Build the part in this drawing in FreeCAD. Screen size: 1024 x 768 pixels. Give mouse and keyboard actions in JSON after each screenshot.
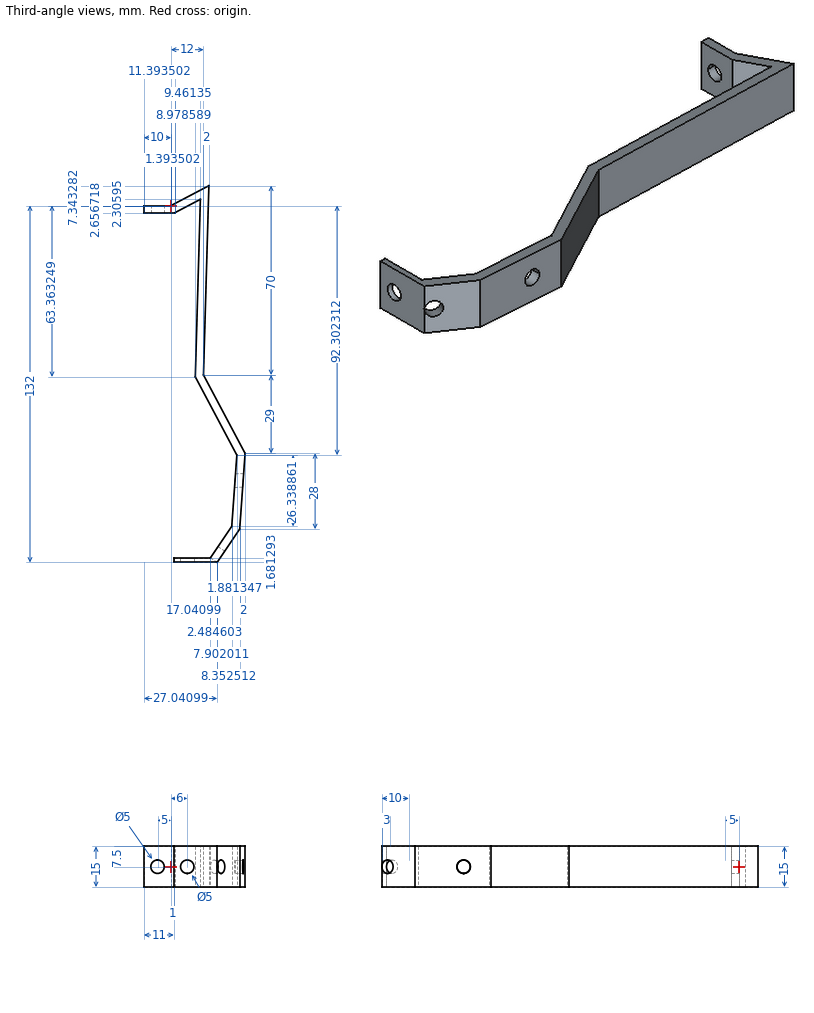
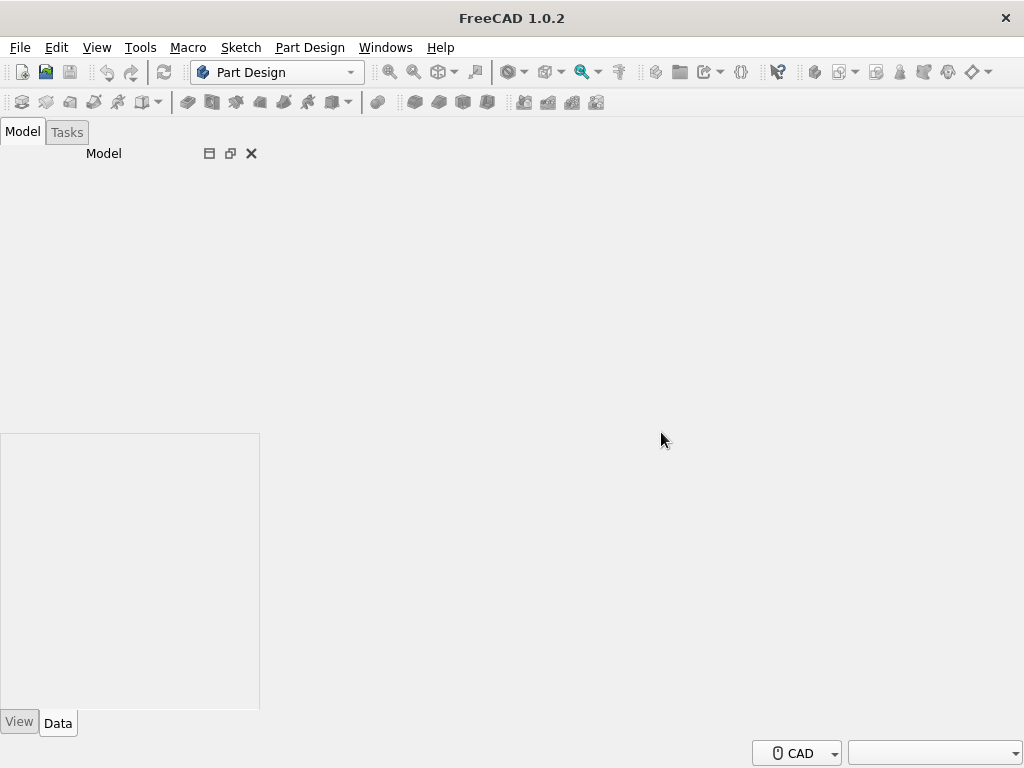
{"action": "left_click", "coordinate": [22, 72]}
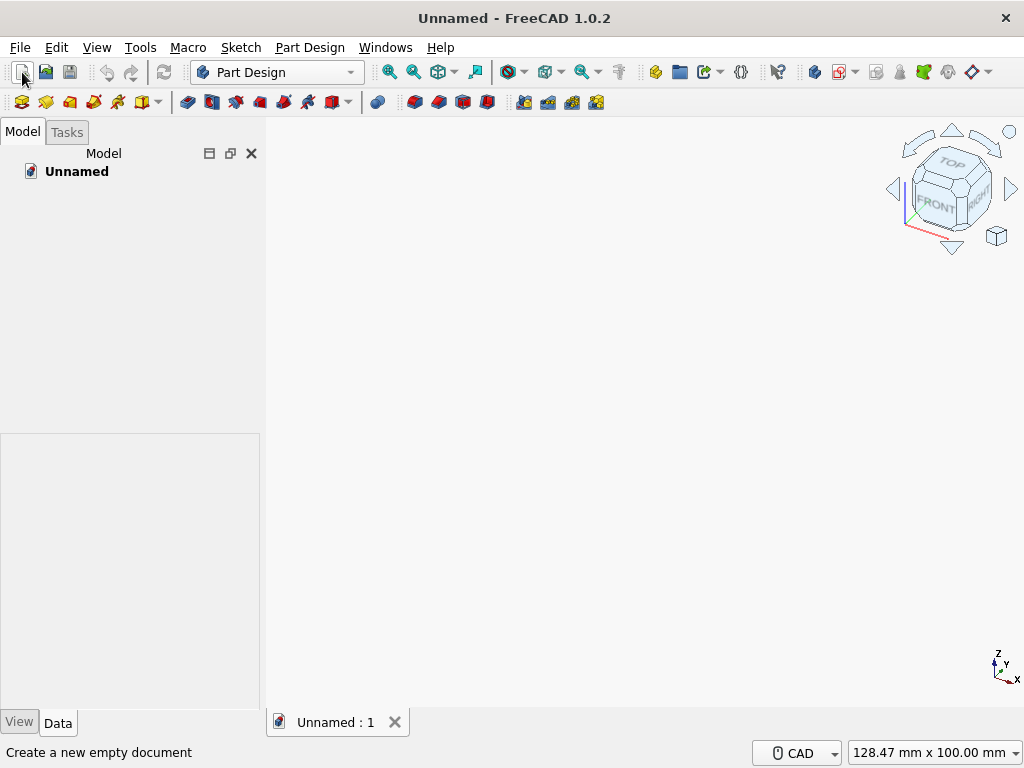
{"action": "left_click", "coordinate": [840, 72]}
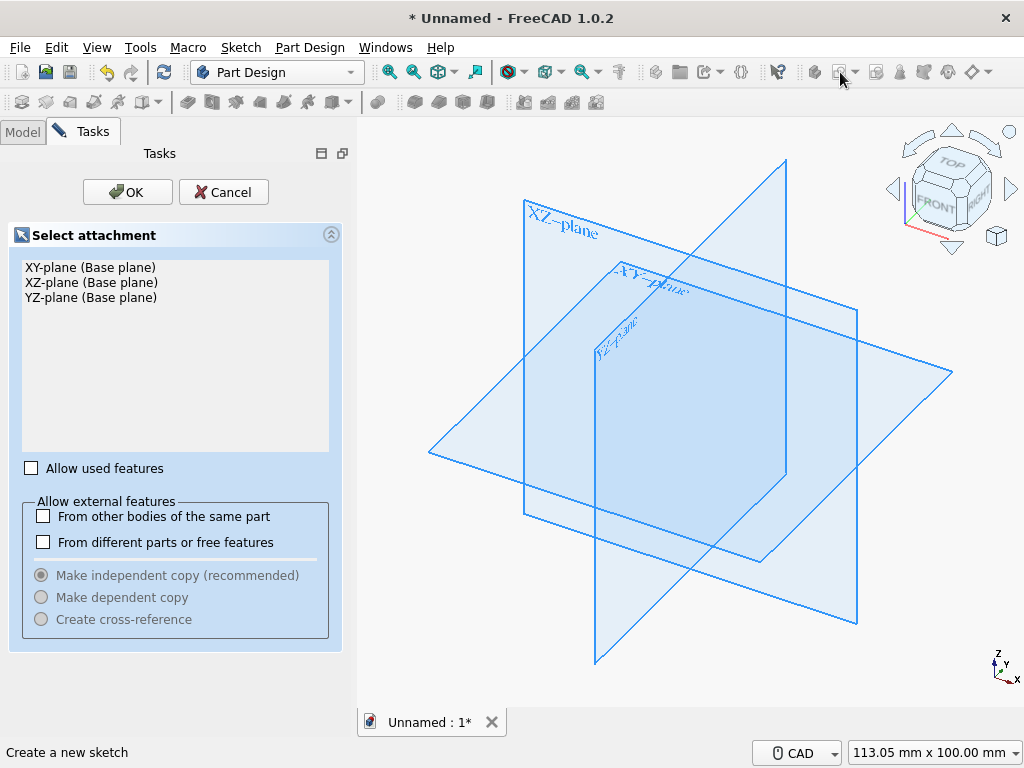
{"action": "left_click", "coordinate": [82, 268]}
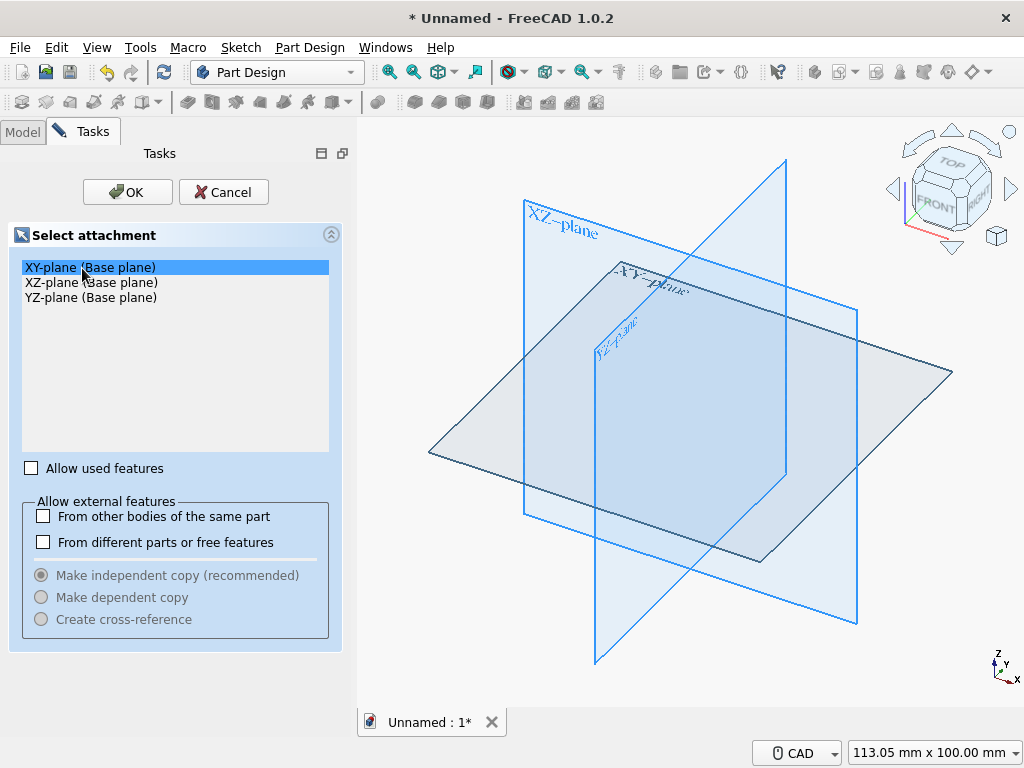
{"action": "left_click", "coordinate": [128, 192]}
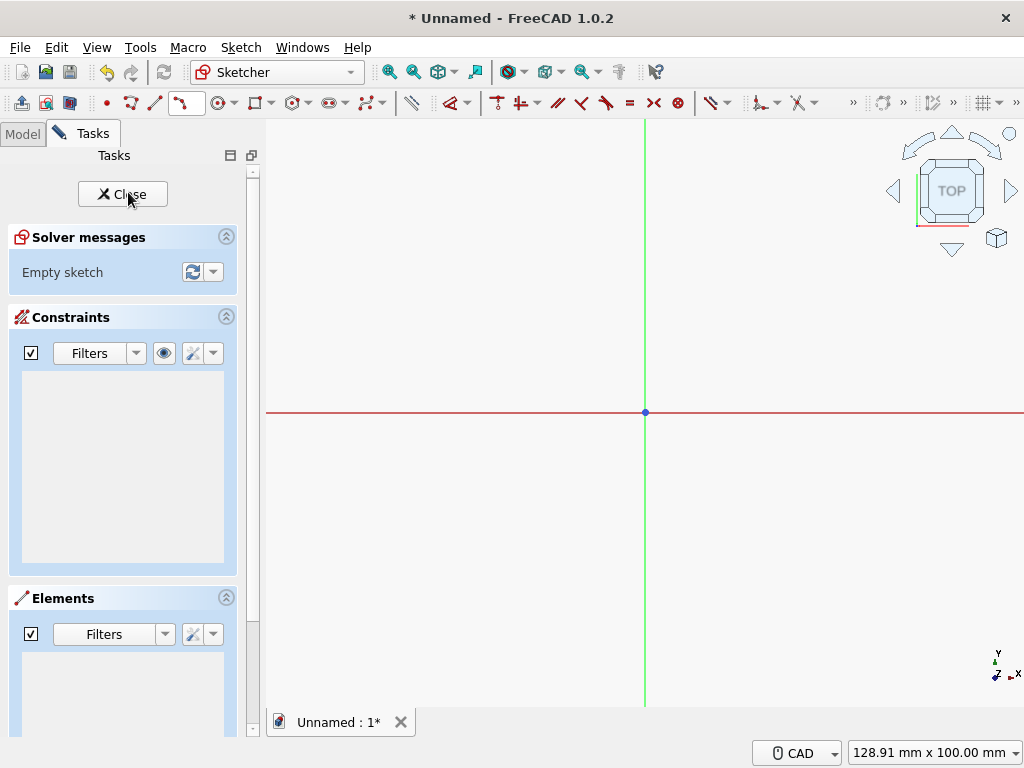
{"action": "scroll", "coordinate": [455, 147], "scroll_direction": "down", "scroll_amount": 4}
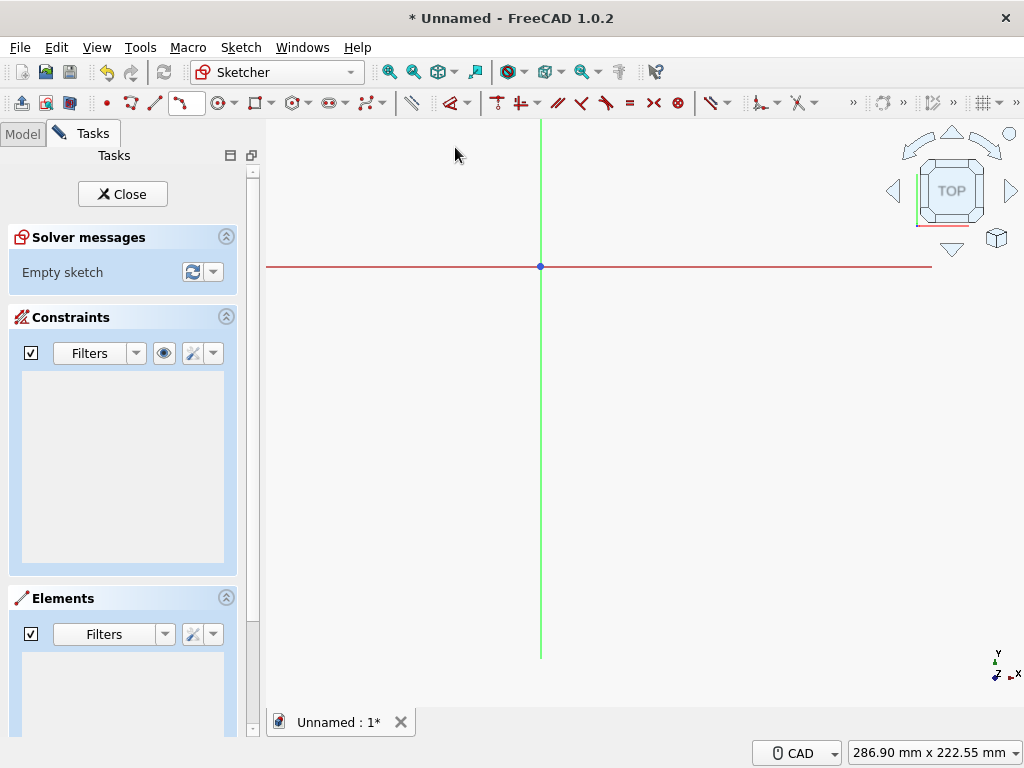
{"action": "left_click", "coordinate": [132, 104]}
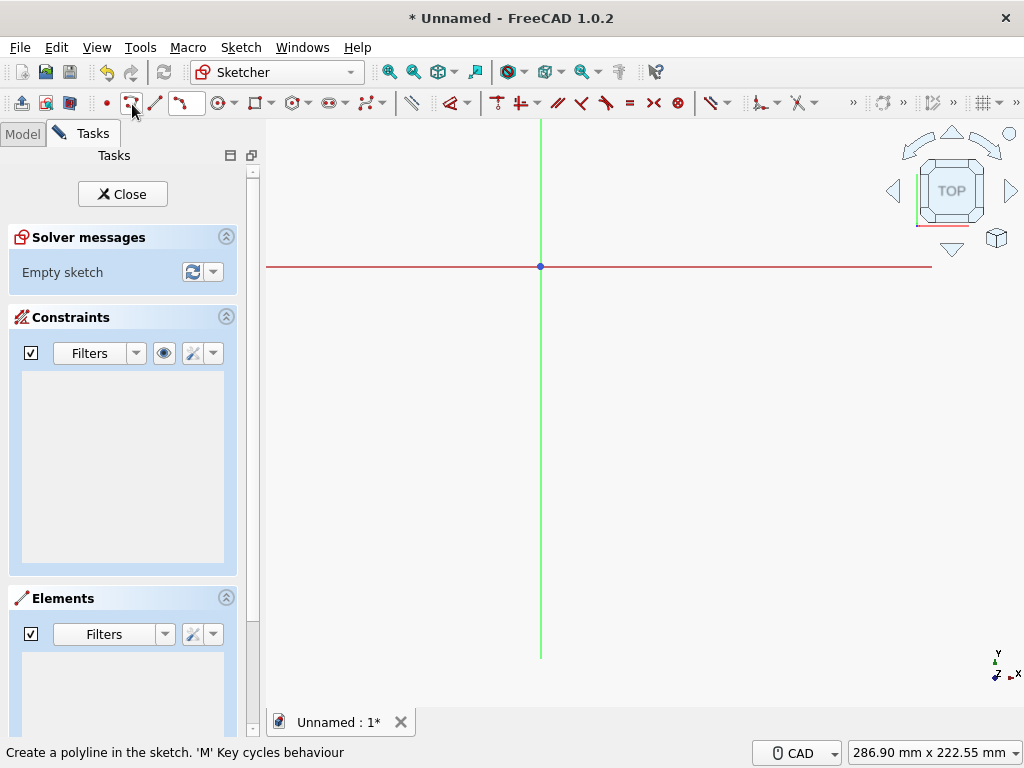
{"action": "left_click", "coordinate": [541, 267]}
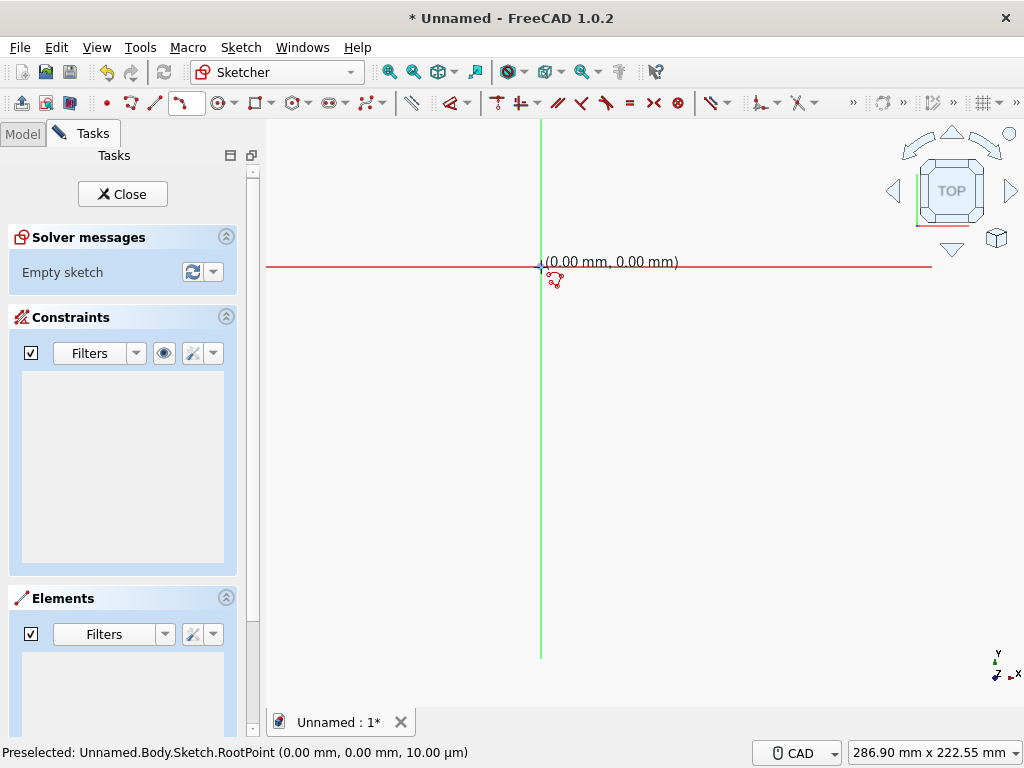
{"action": "scroll", "coordinate": [544, 274], "scroll_direction": "up", "scroll_amount": 8}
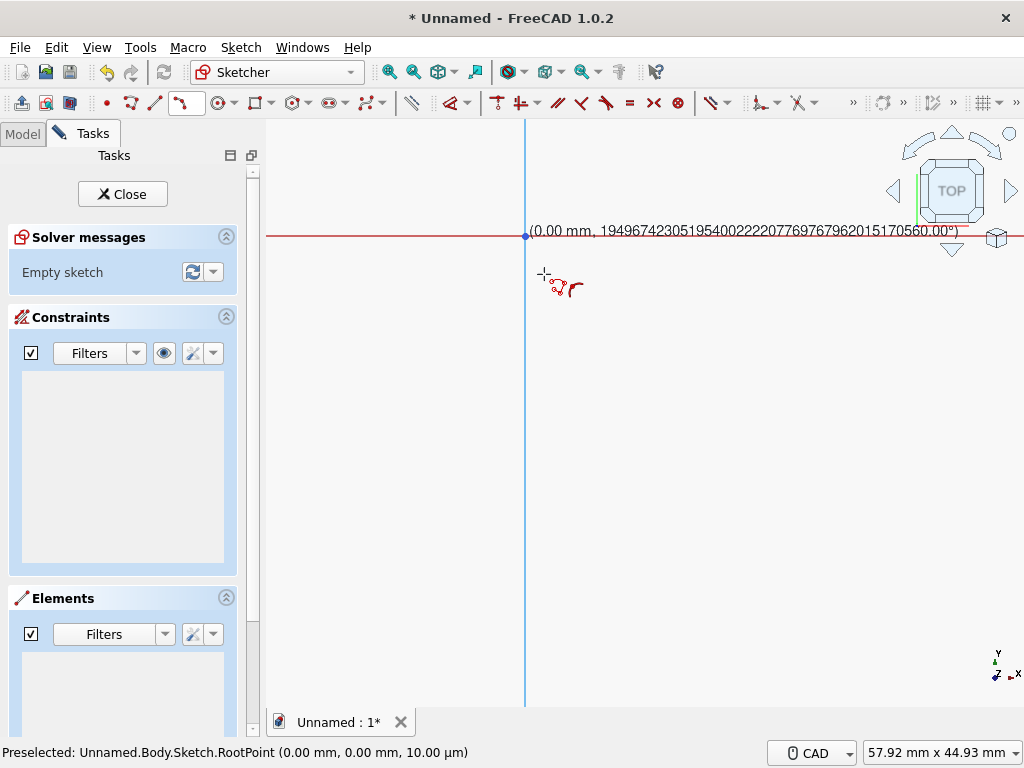
{"action": "left_click", "coordinate": [543, 271]}
{"action": "left_click", "coordinate": [667, 206]}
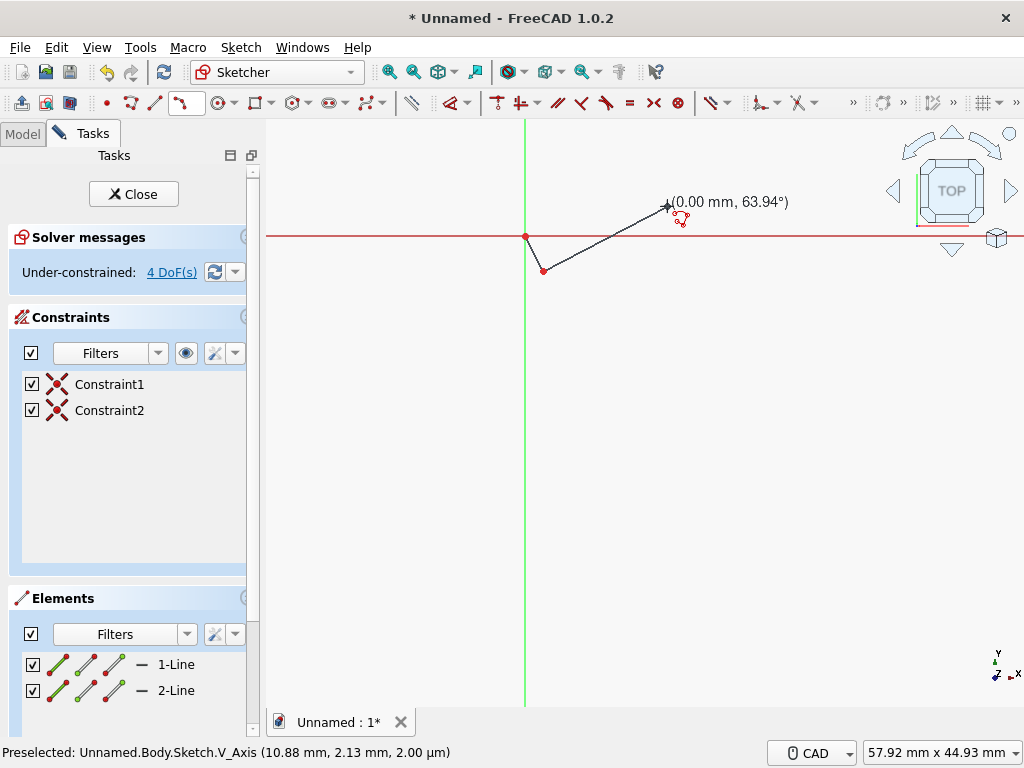
{"action": "scroll", "coordinate": [544, 251], "scroll_direction": "down", "scroll_amount": 8}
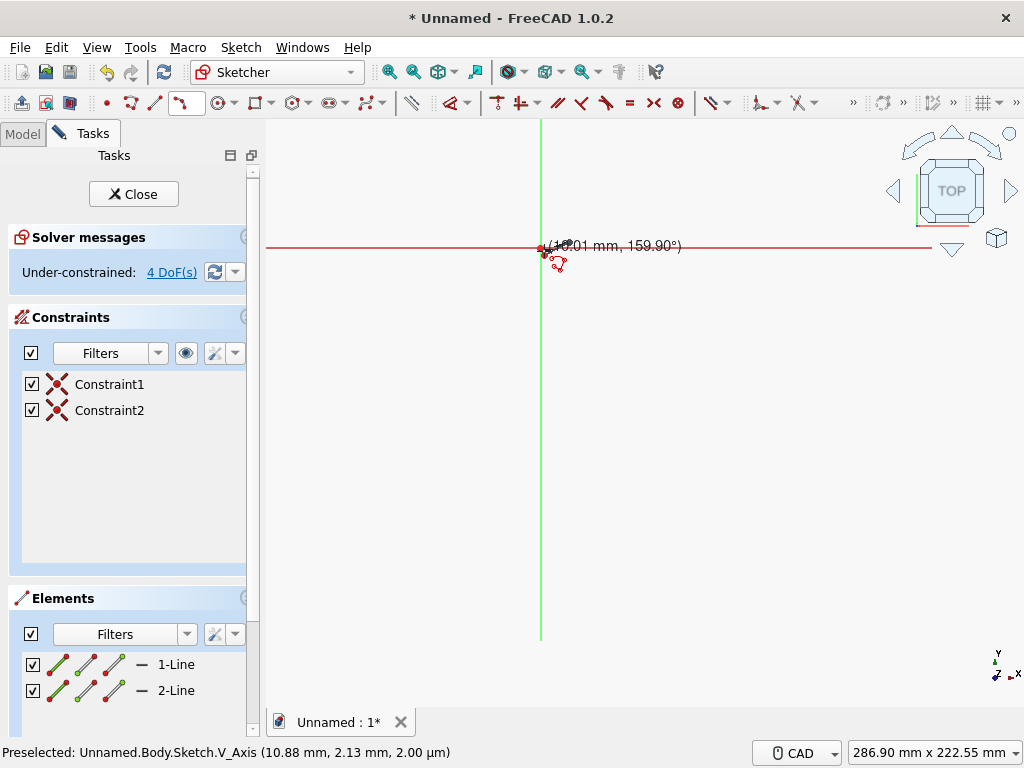
{"action": "left_click", "coordinate": [560, 416]}
{"action": "left_click", "coordinate": [605, 492]}
{"action": "left_click", "coordinate": [600, 562]}
{"action": "left_click", "coordinate": [579, 592]}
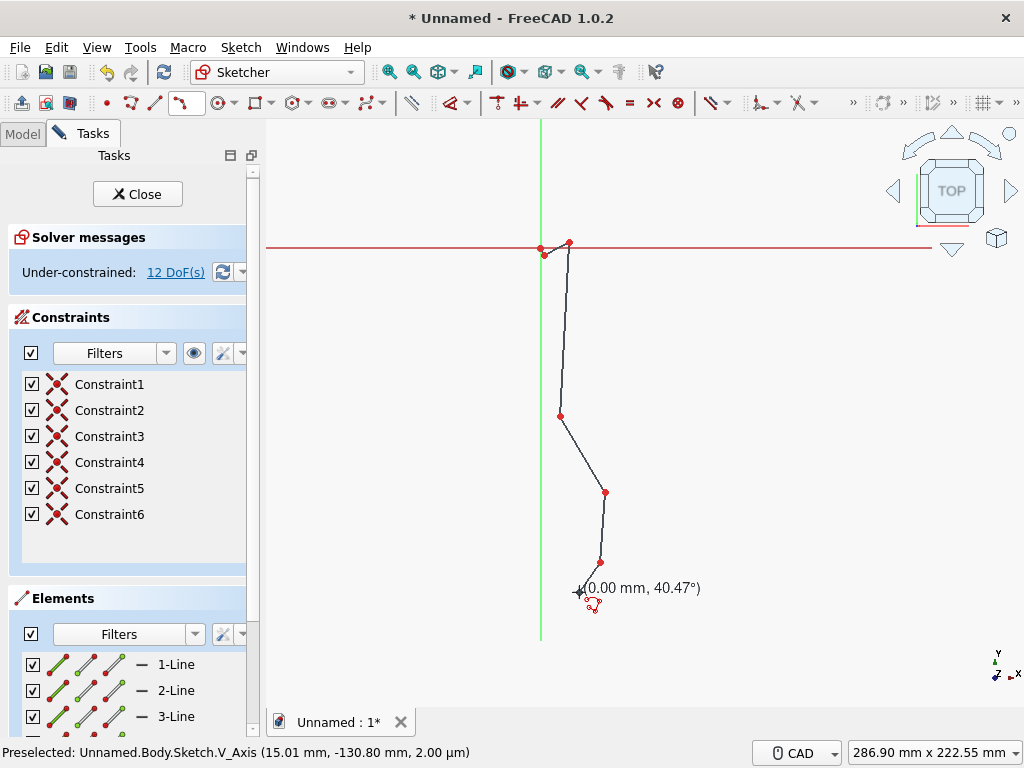
{"action": "scroll", "coordinate": [586, 597], "scroll_direction": "up", "scroll_amount": 4}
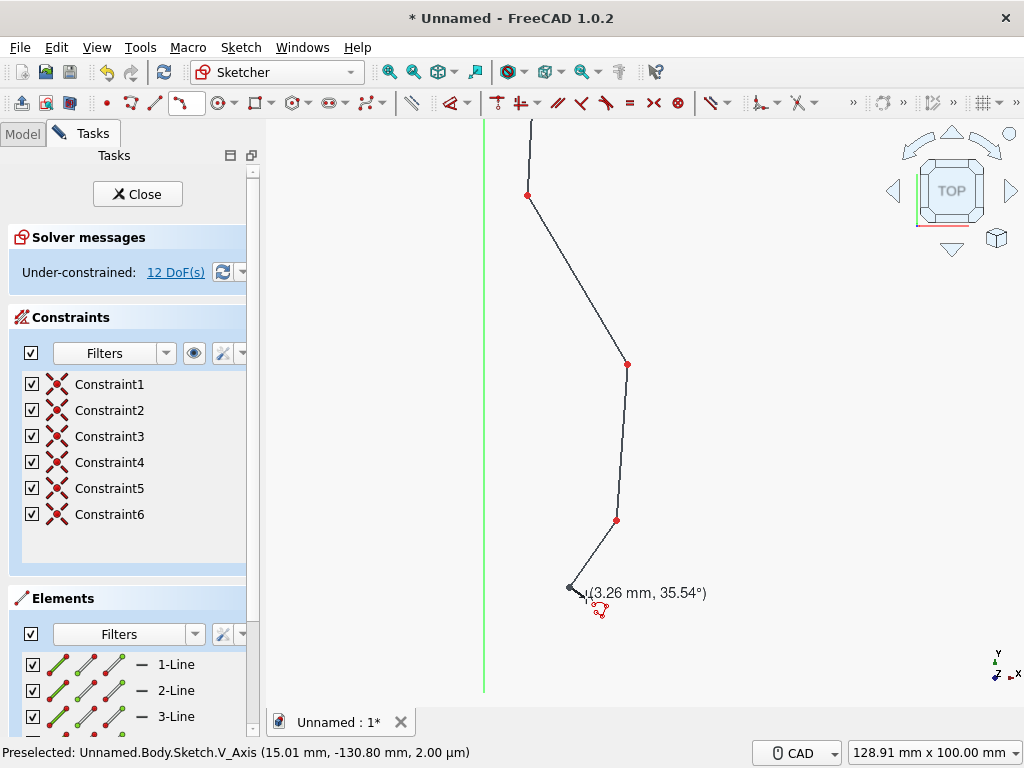
{"action": "left_click", "coordinate": [584, 596]}
{"action": "left_click", "coordinate": [634, 523]}
{"action": "left_click", "coordinate": [645, 359]}
{"action": "left_click", "coordinate": [555, 188]}